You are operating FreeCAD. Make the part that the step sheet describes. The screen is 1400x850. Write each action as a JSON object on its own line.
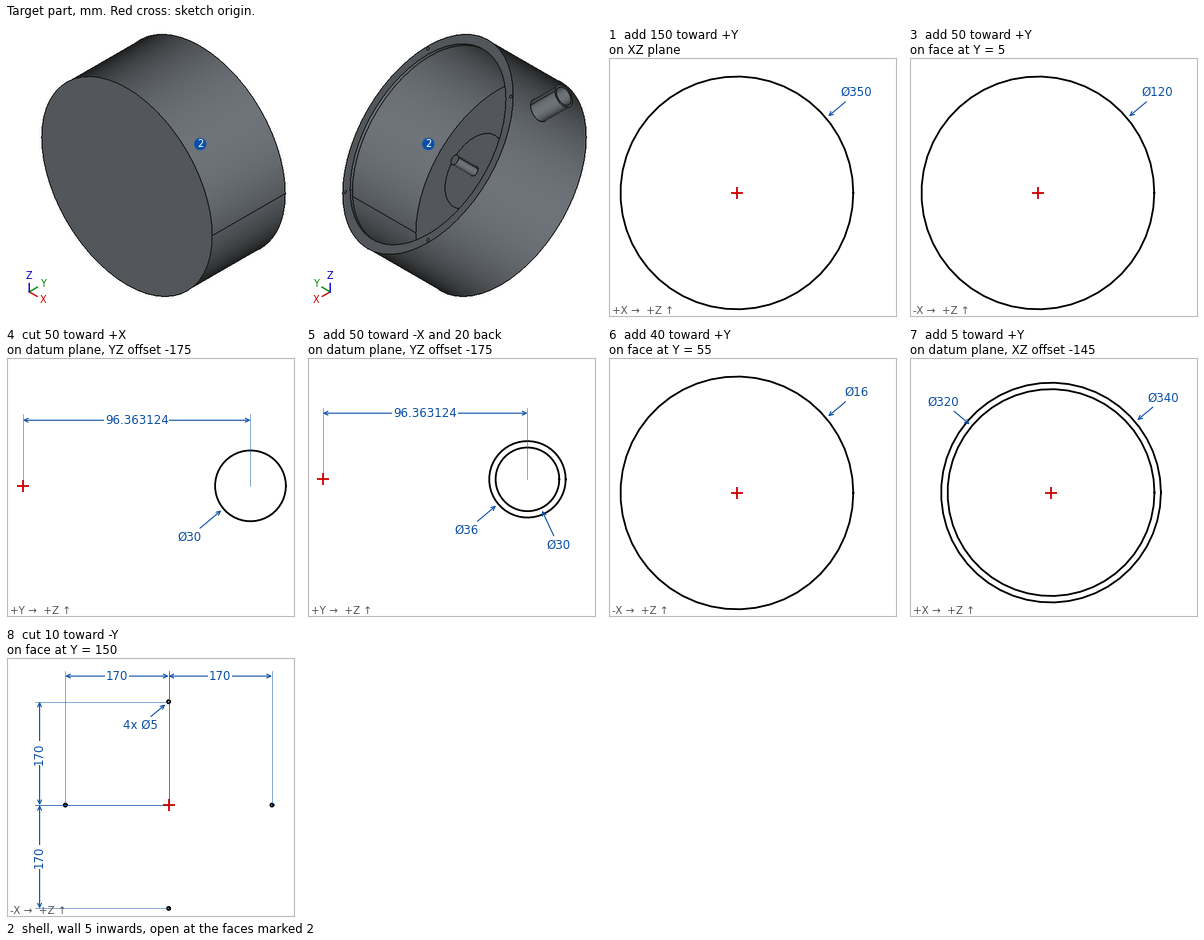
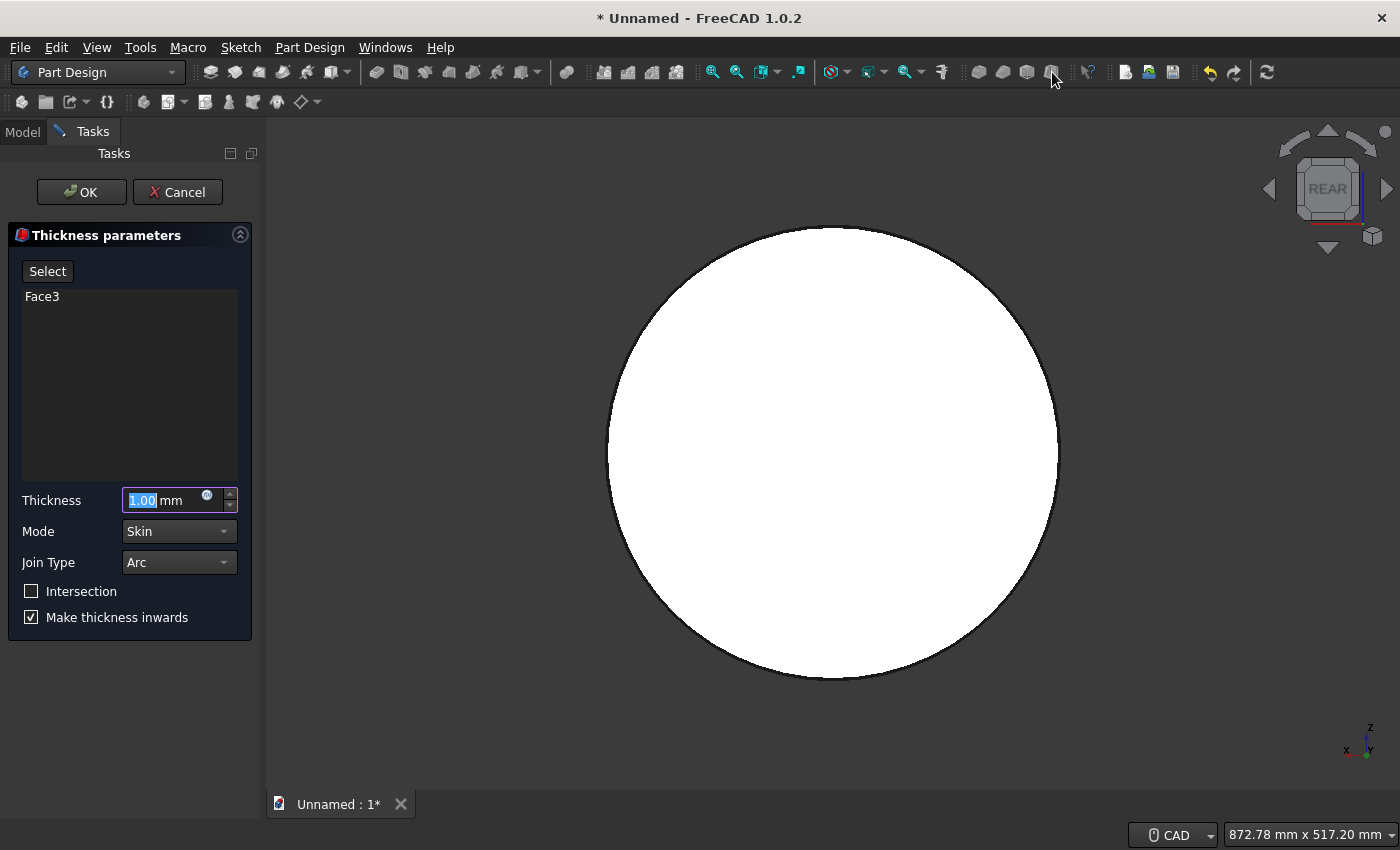
{"action": "type", "text": "5"}
{"action": "key", "text": "Tab"}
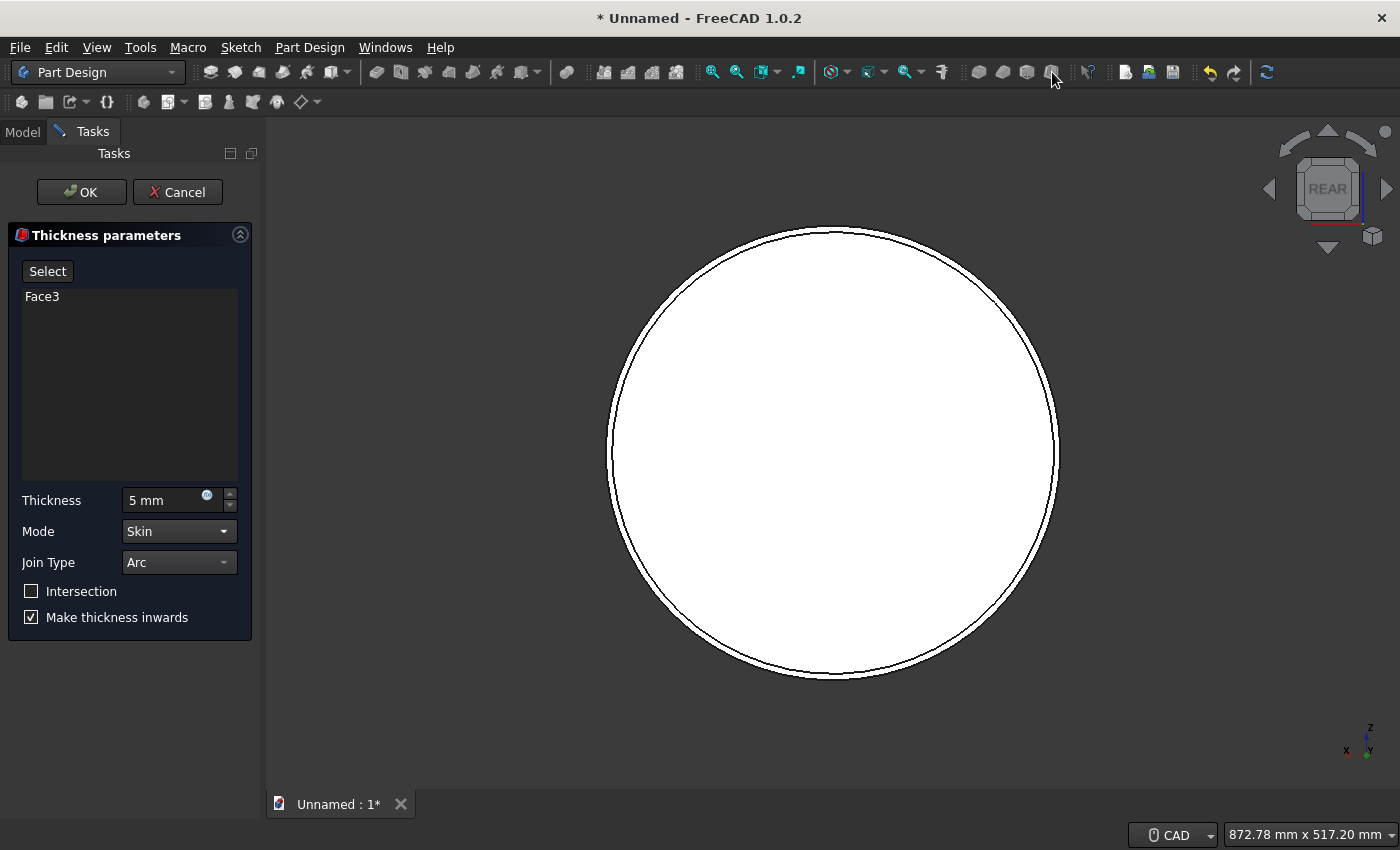
{"action": "left_click", "coordinate": [180, 562]}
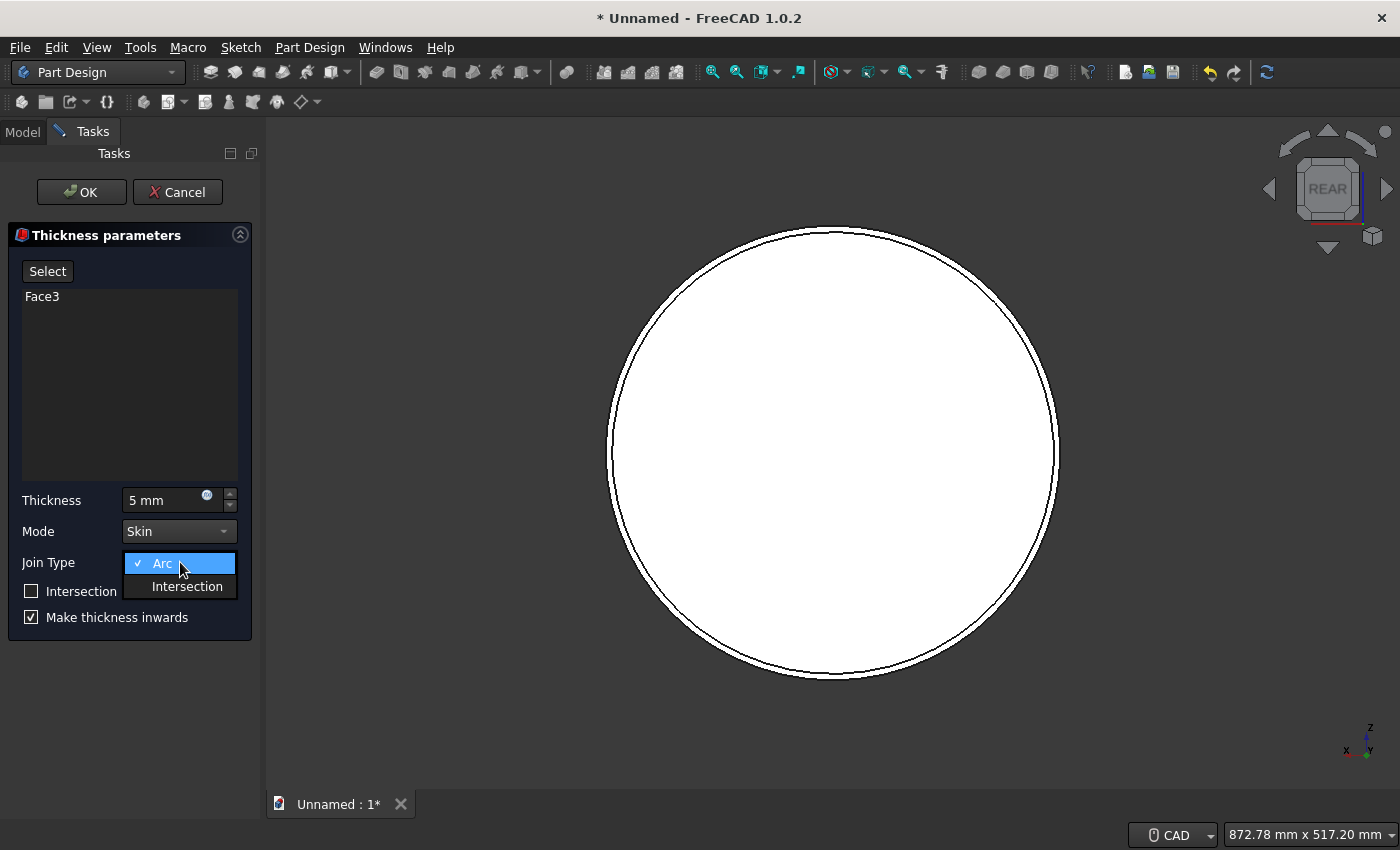
{"action": "left_click", "coordinate": [179, 586]}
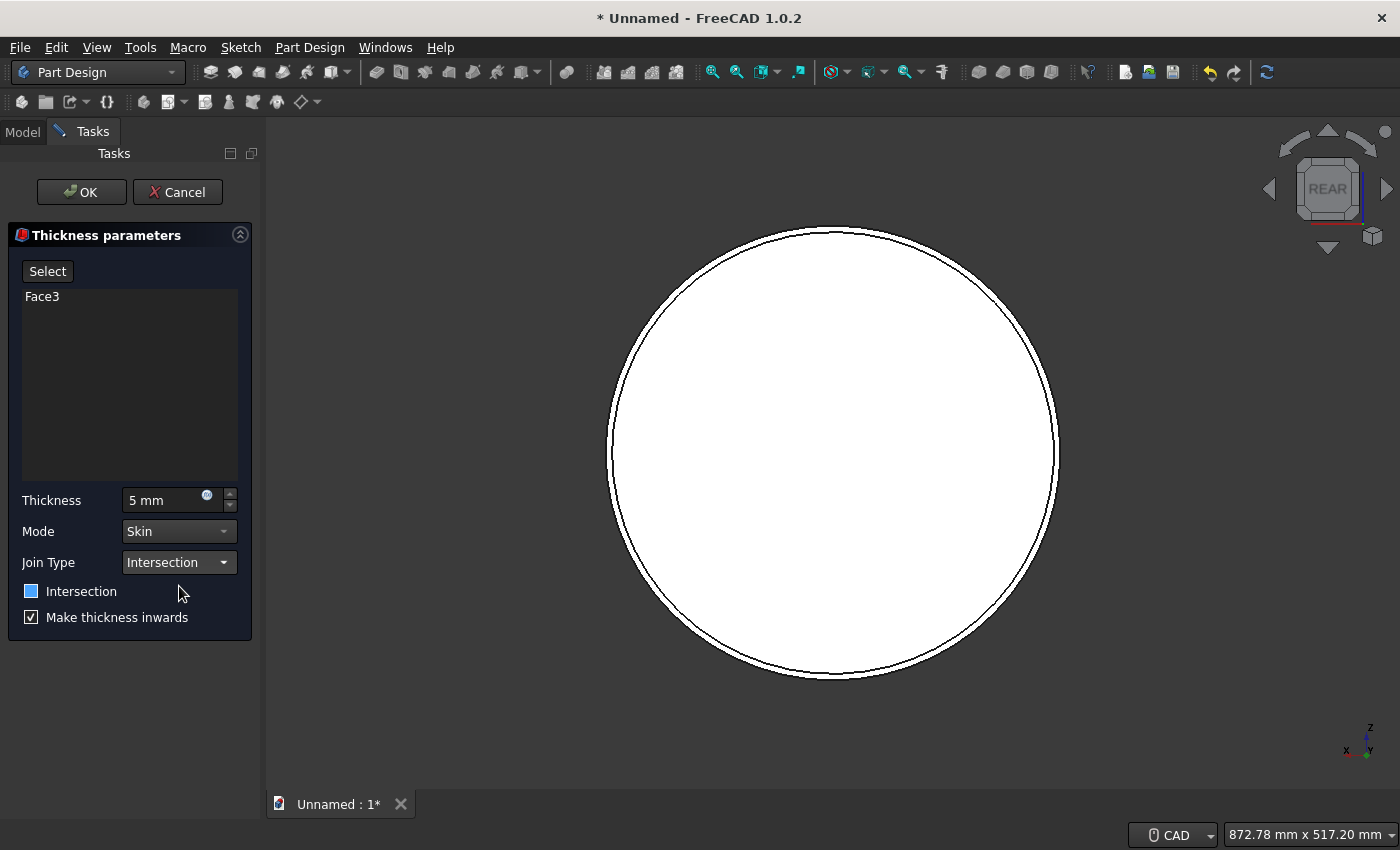
{"action": "left_click", "coordinate": [82, 192]}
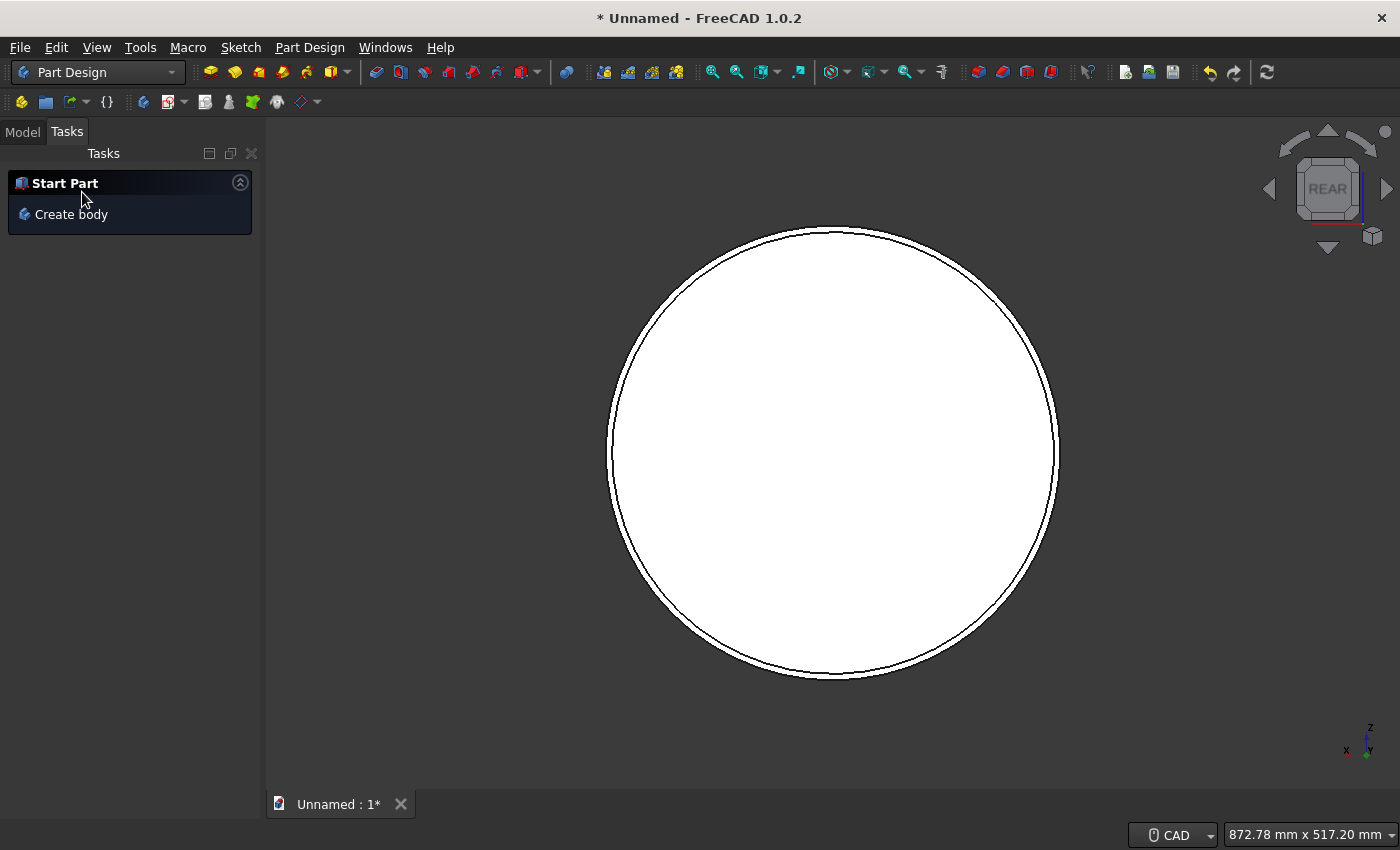
{"action": "left_click", "coordinate": [833, 452]}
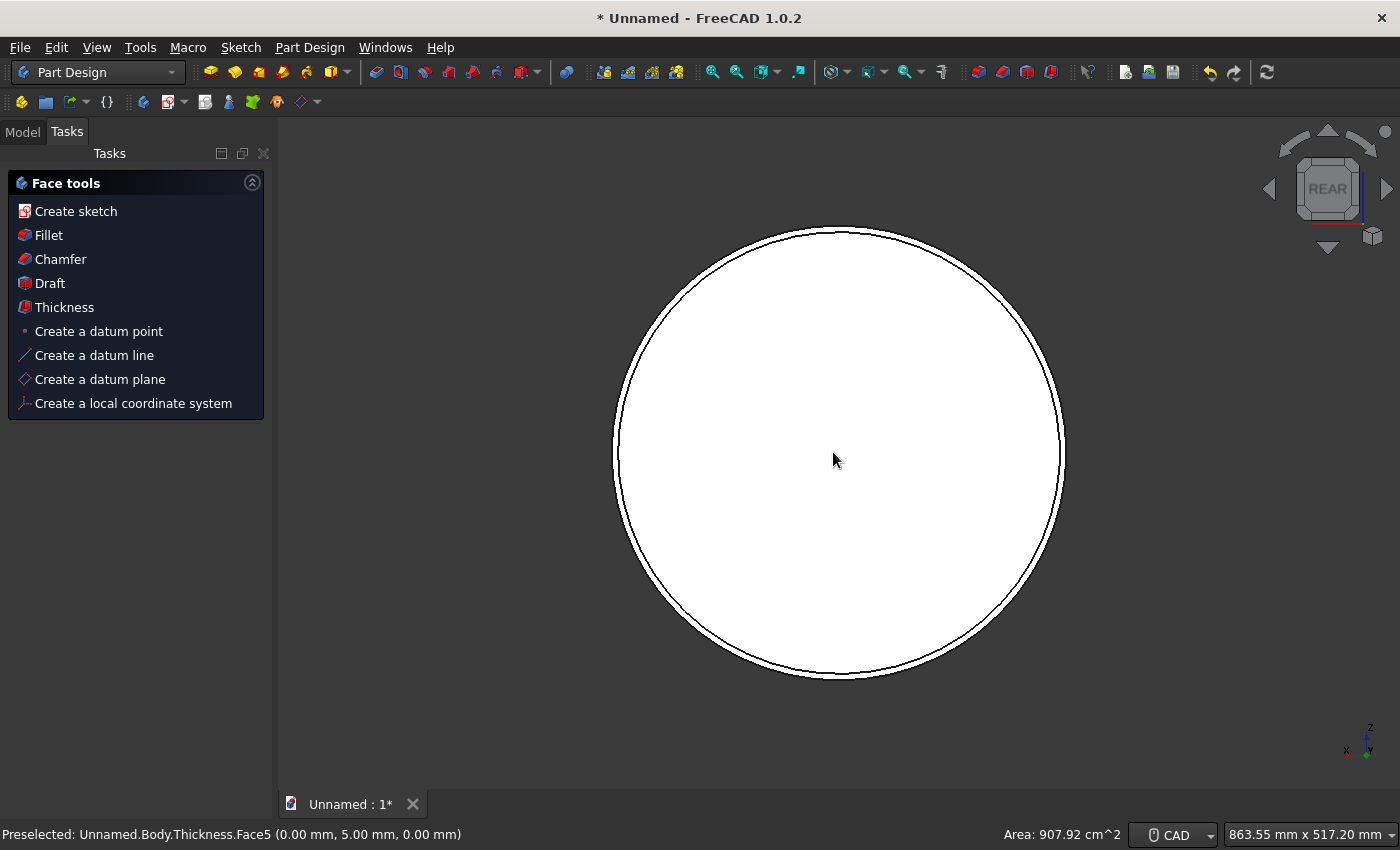
{"action": "left_click", "coordinate": [168, 102]}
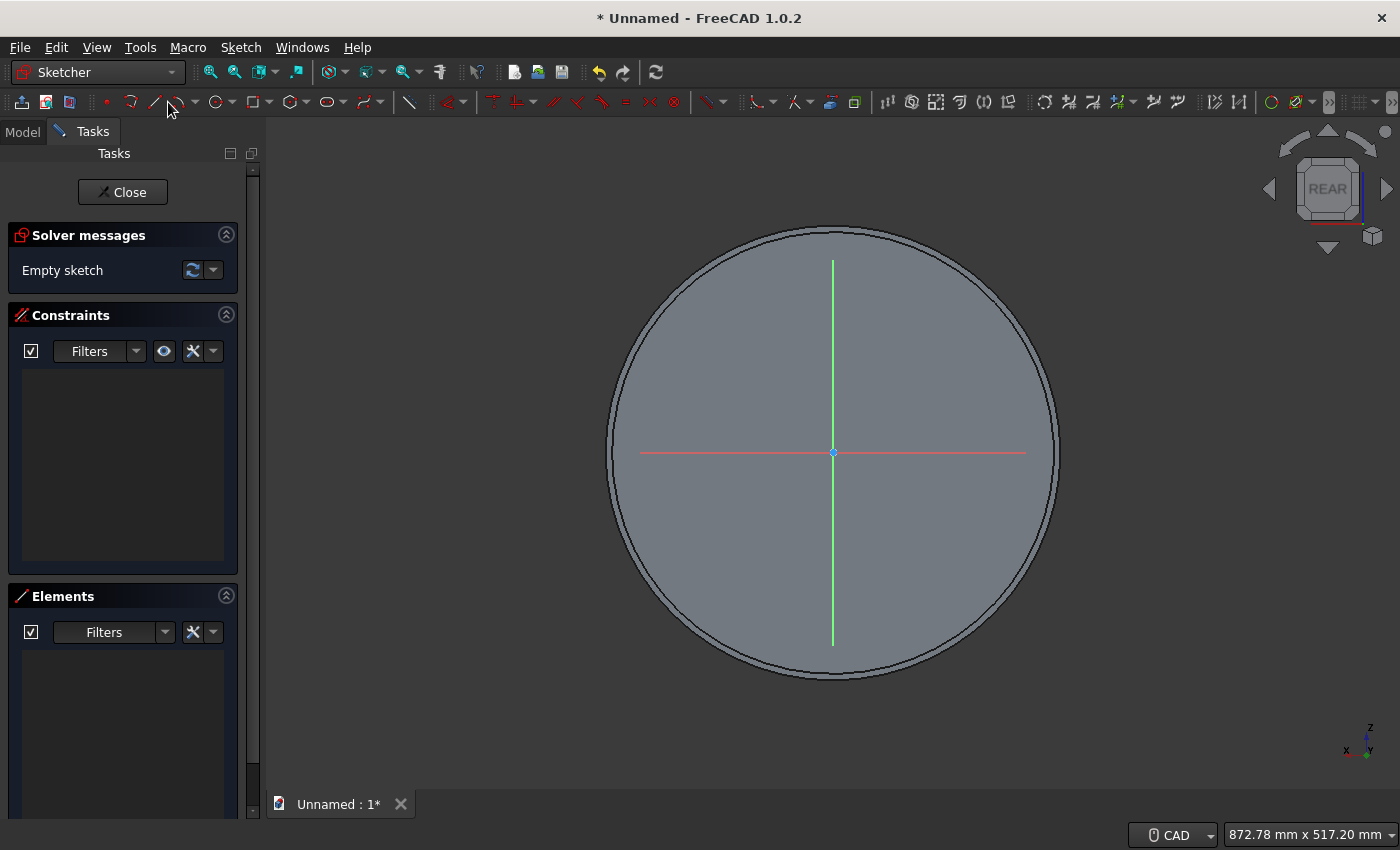
{"action": "scroll", "coordinate": [873, 453], "scroll_direction": "up", "scroll_amount": 5}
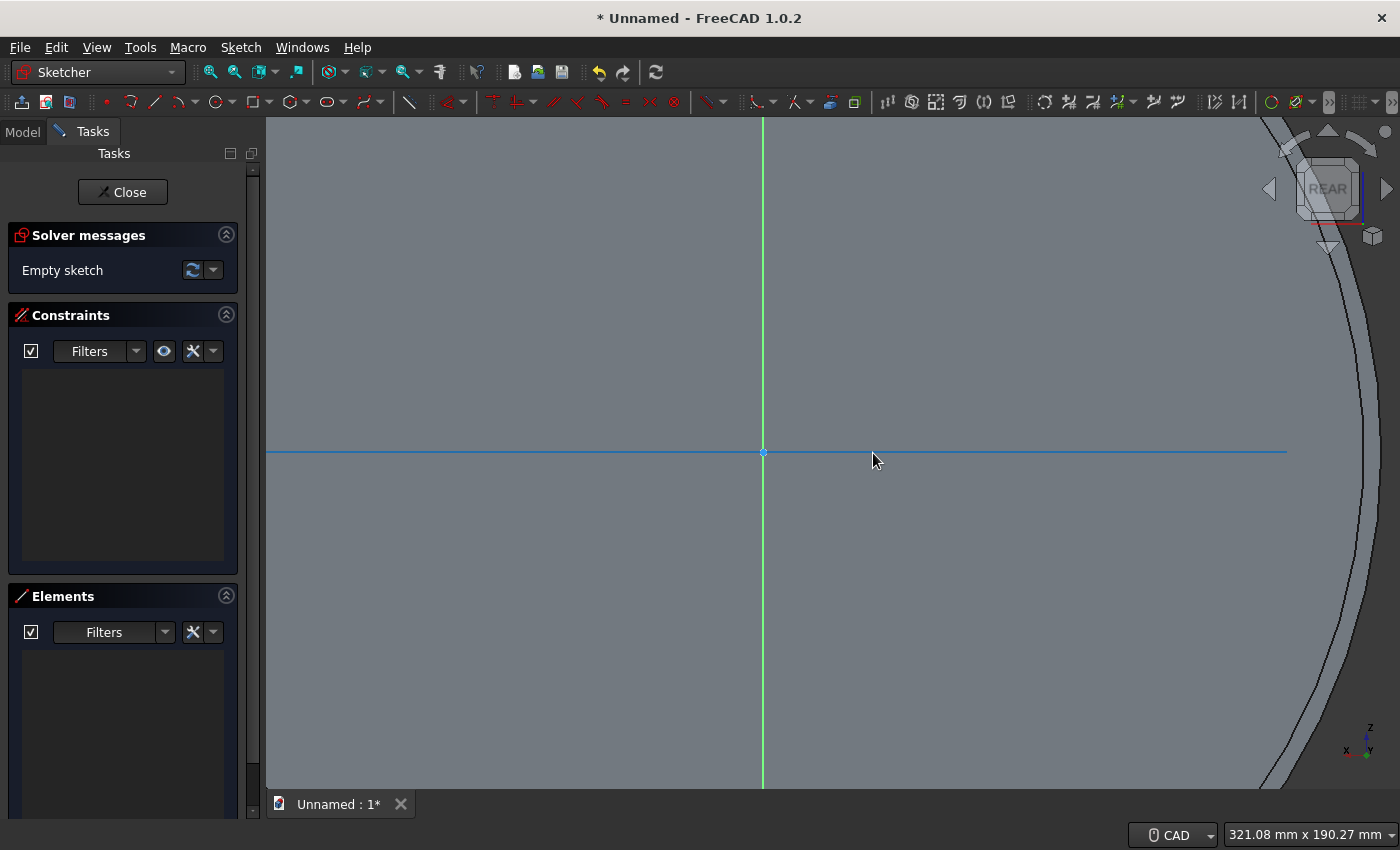
{"action": "left_click", "coordinate": [216, 102]}